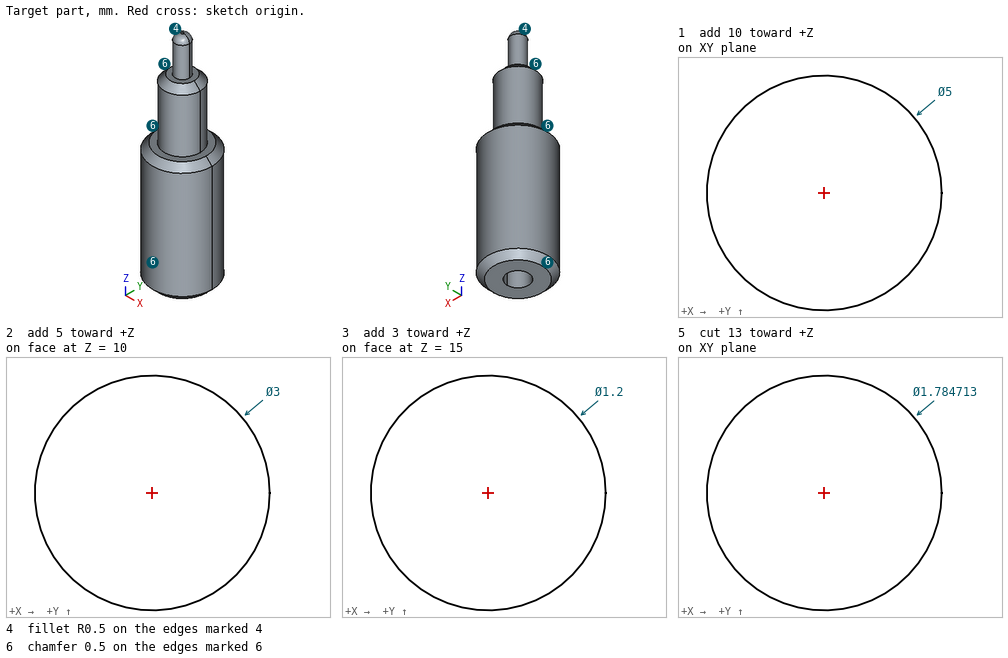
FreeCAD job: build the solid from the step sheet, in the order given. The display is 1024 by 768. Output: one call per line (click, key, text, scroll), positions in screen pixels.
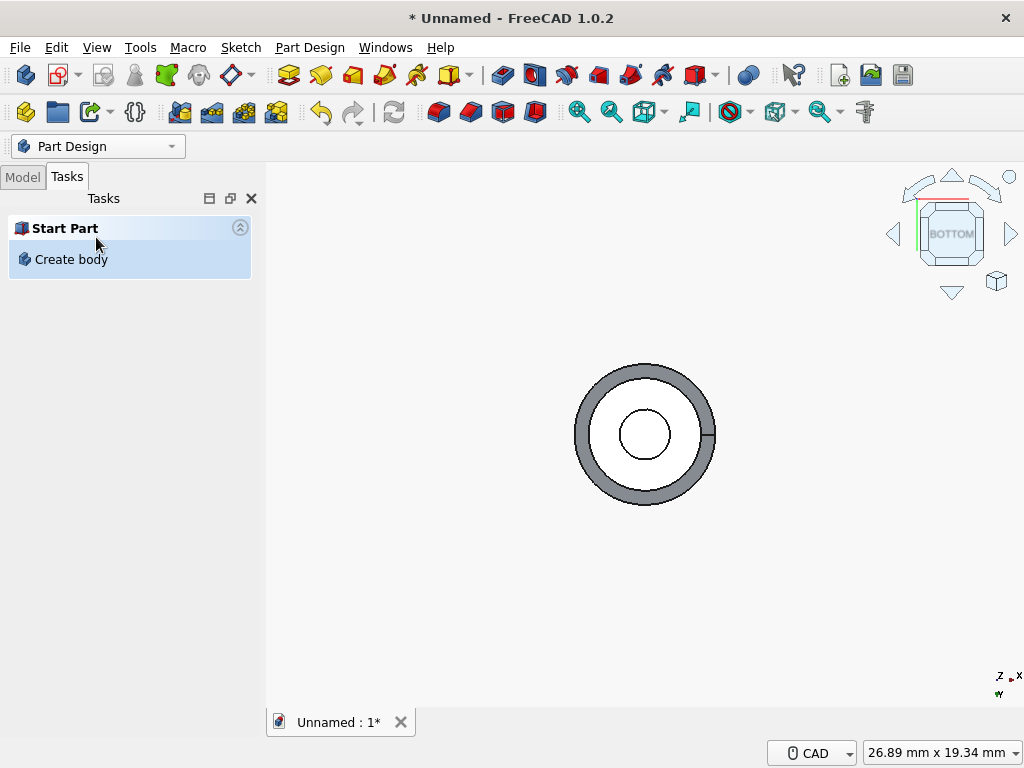
key(0)